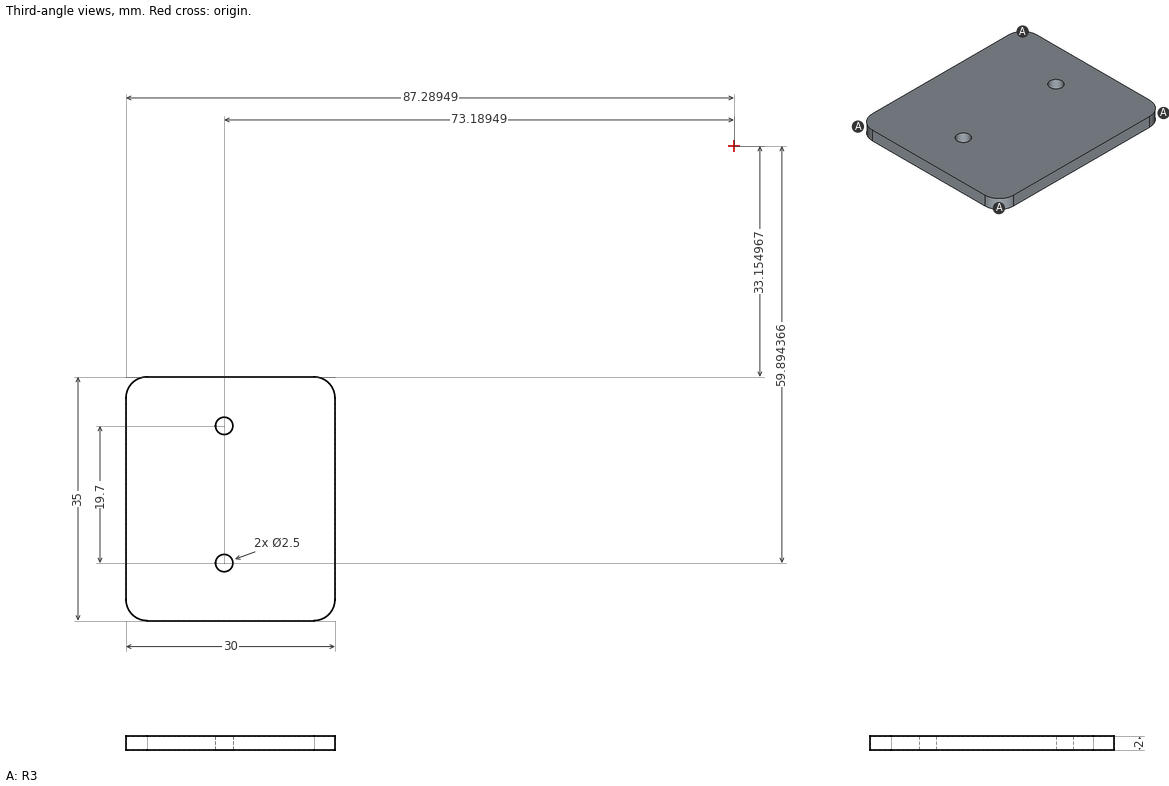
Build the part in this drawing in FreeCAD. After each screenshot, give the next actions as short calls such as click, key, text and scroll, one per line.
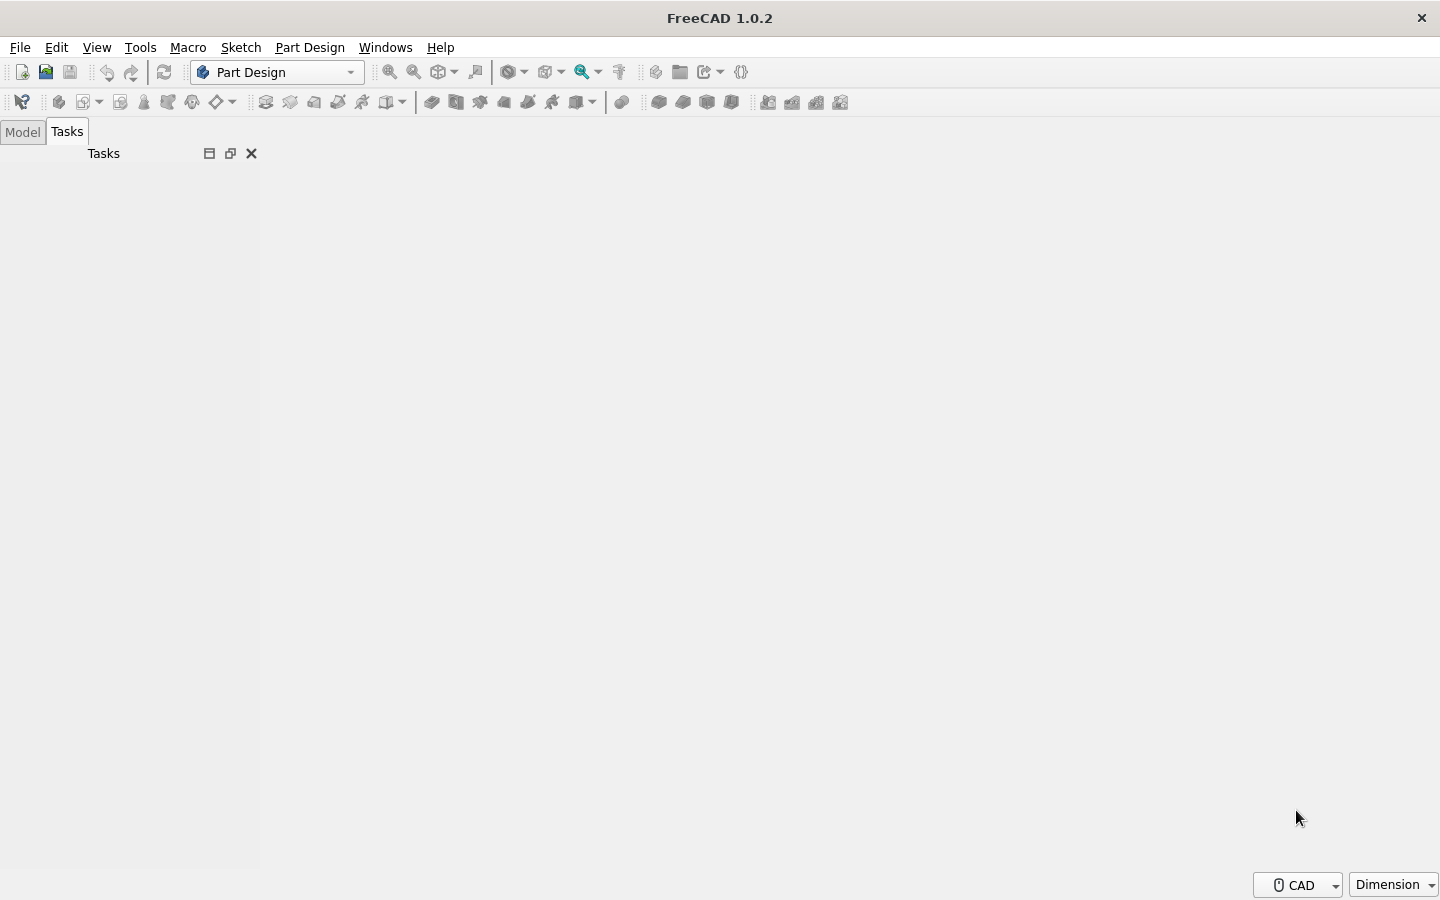
click(22, 72)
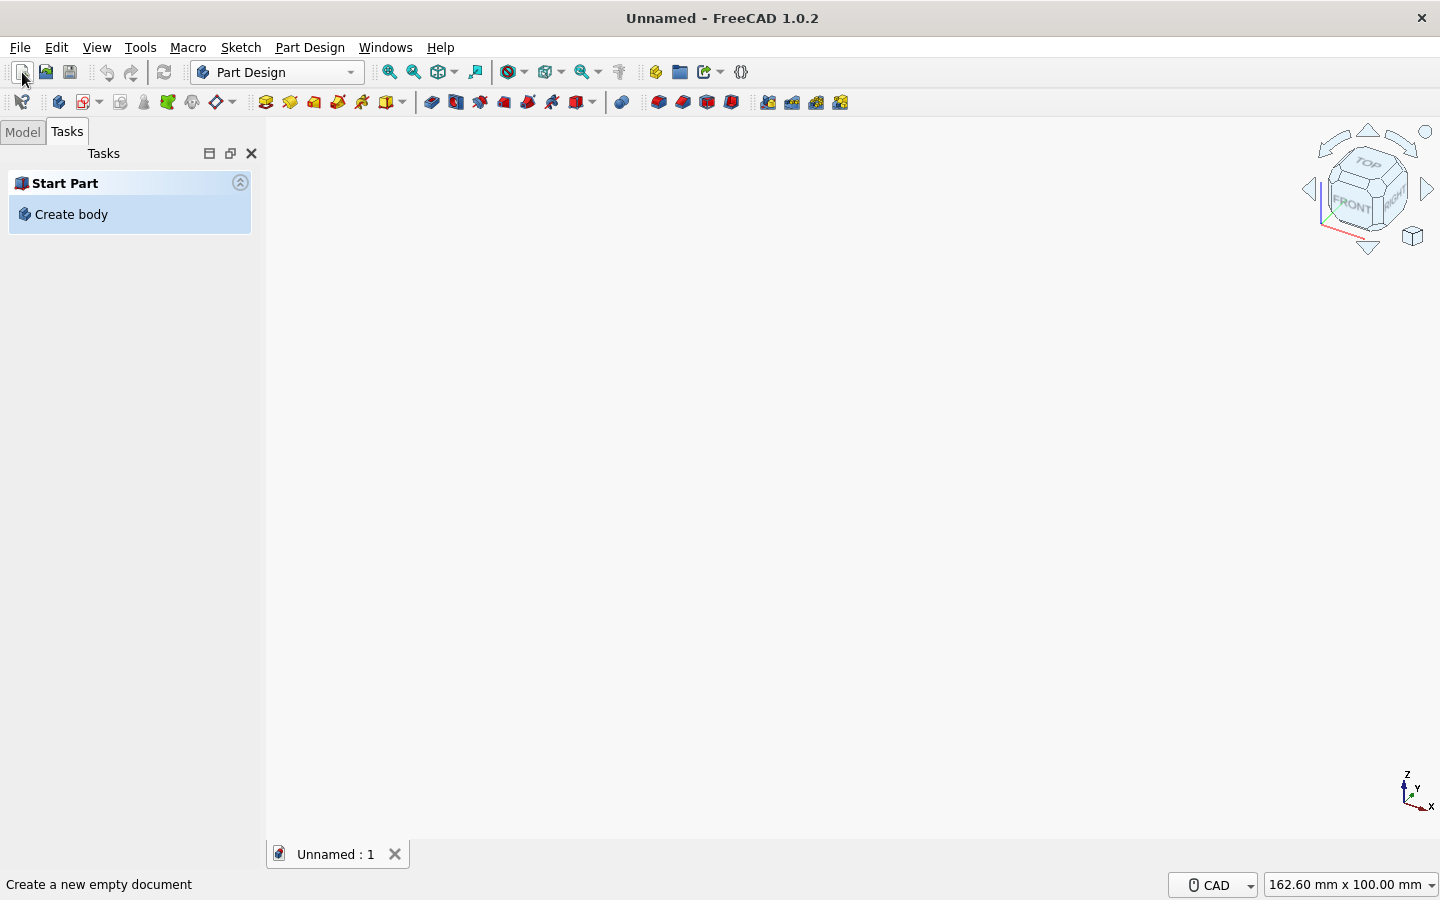
click(84, 102)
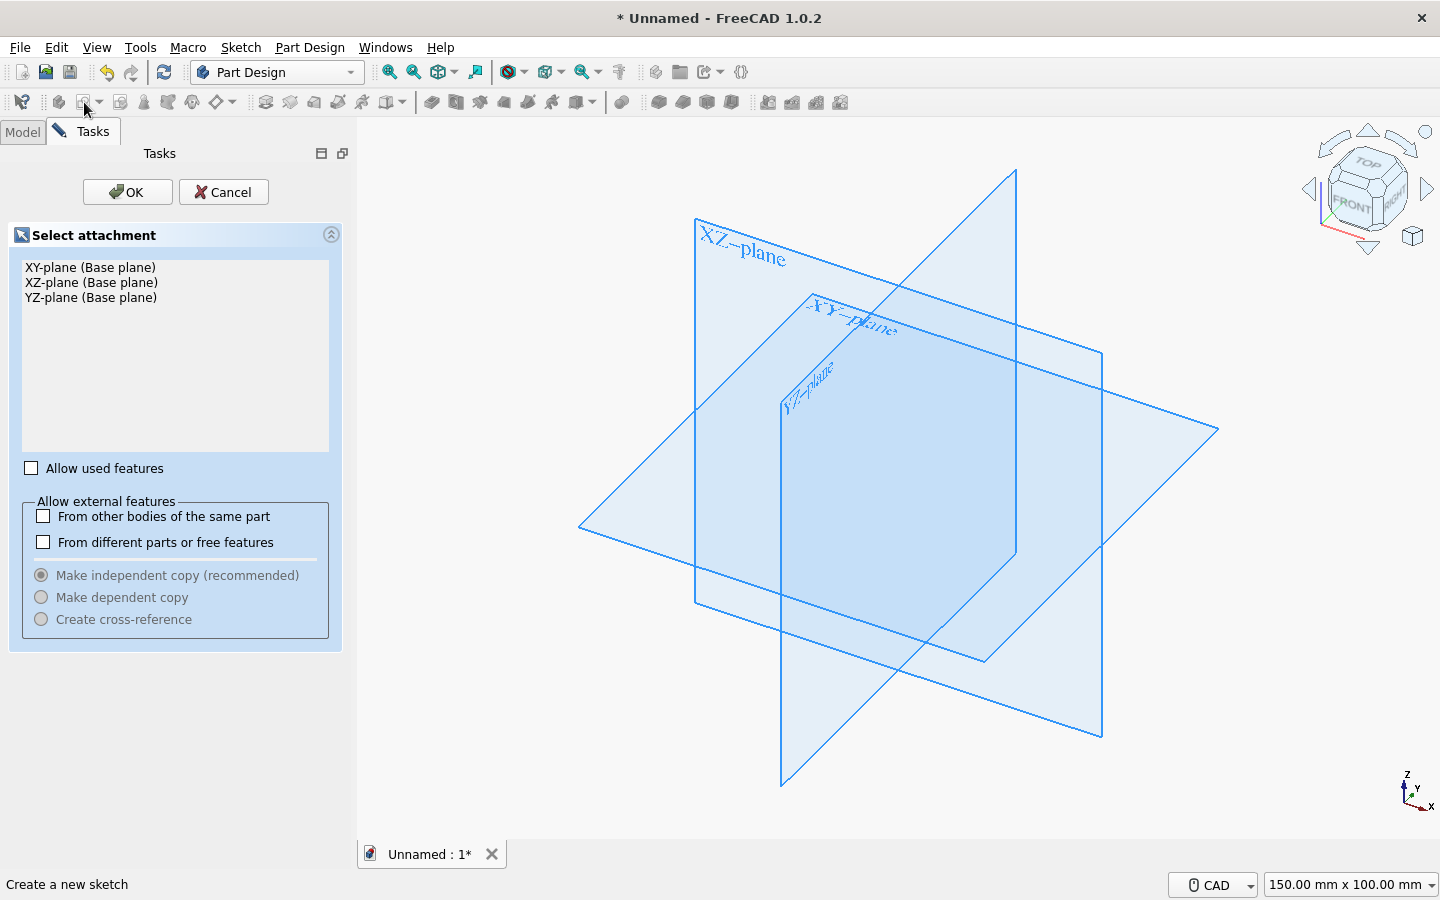
click(82, 268)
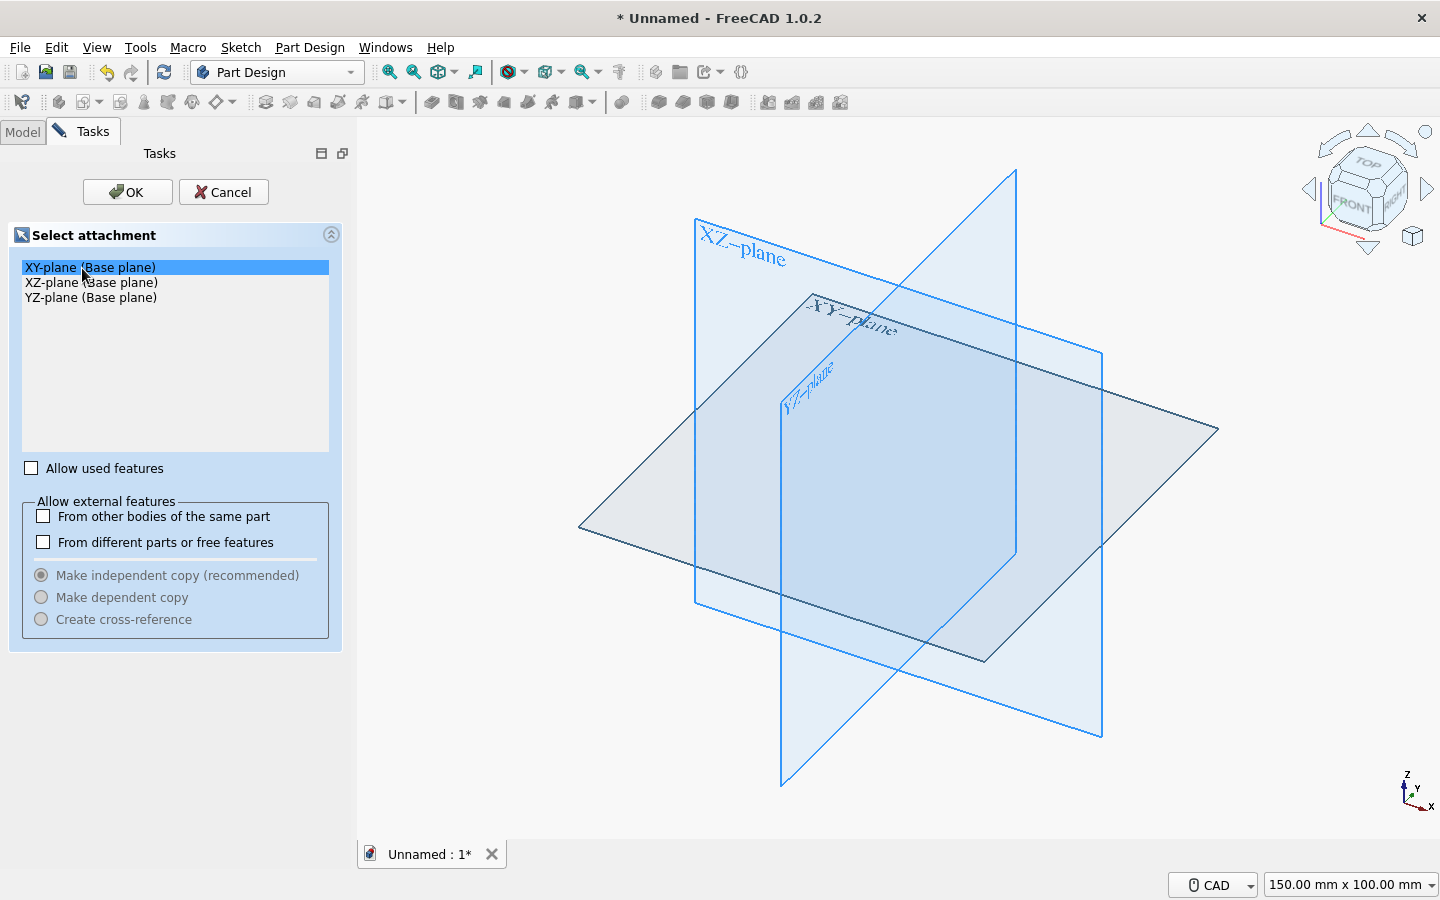
click(128, 192)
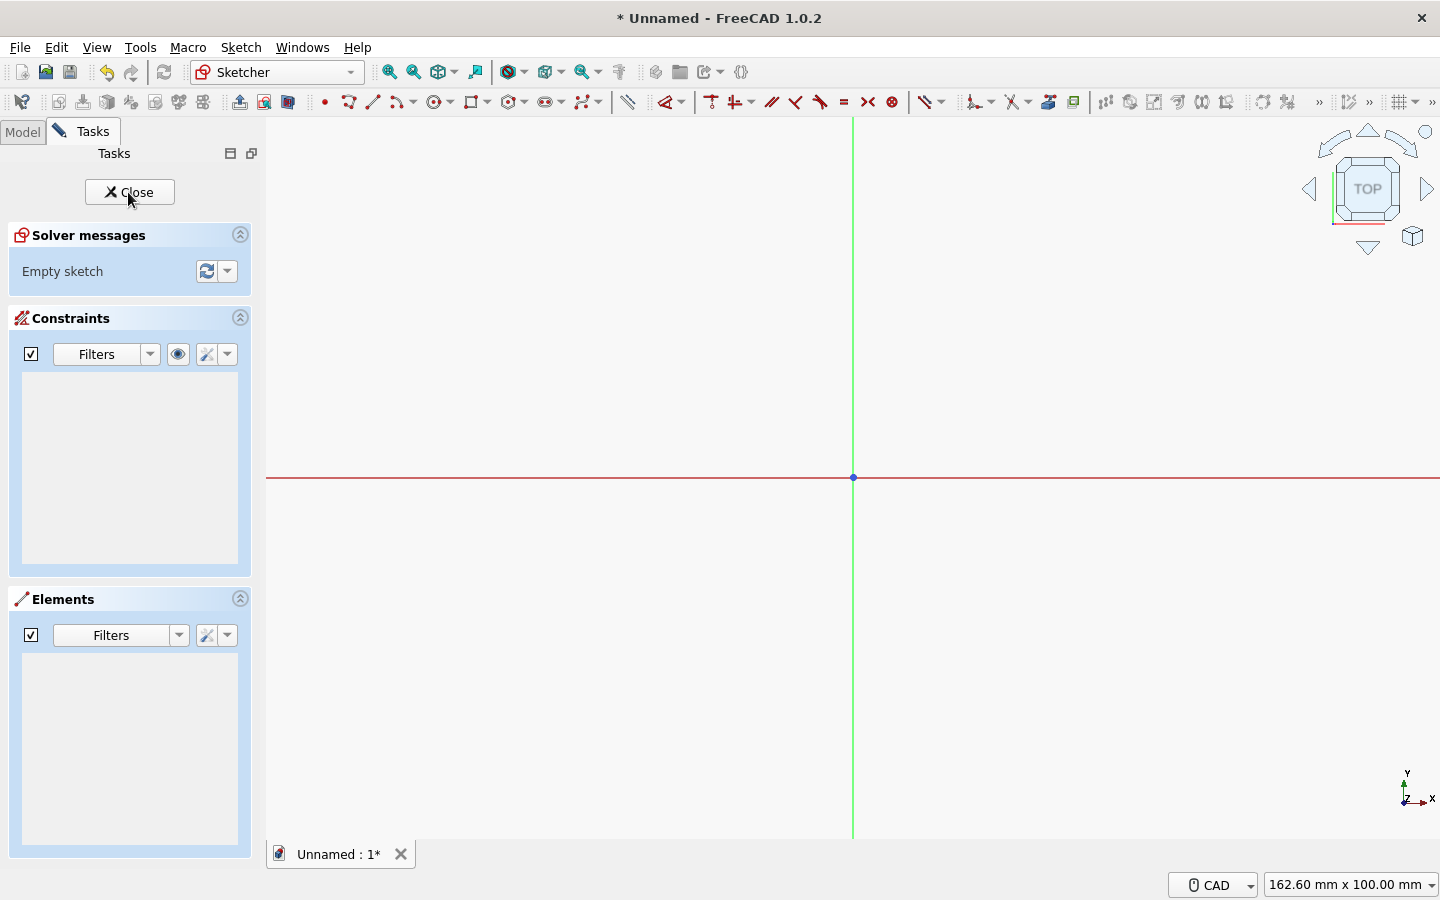
scroll(1275, 145, down, 2)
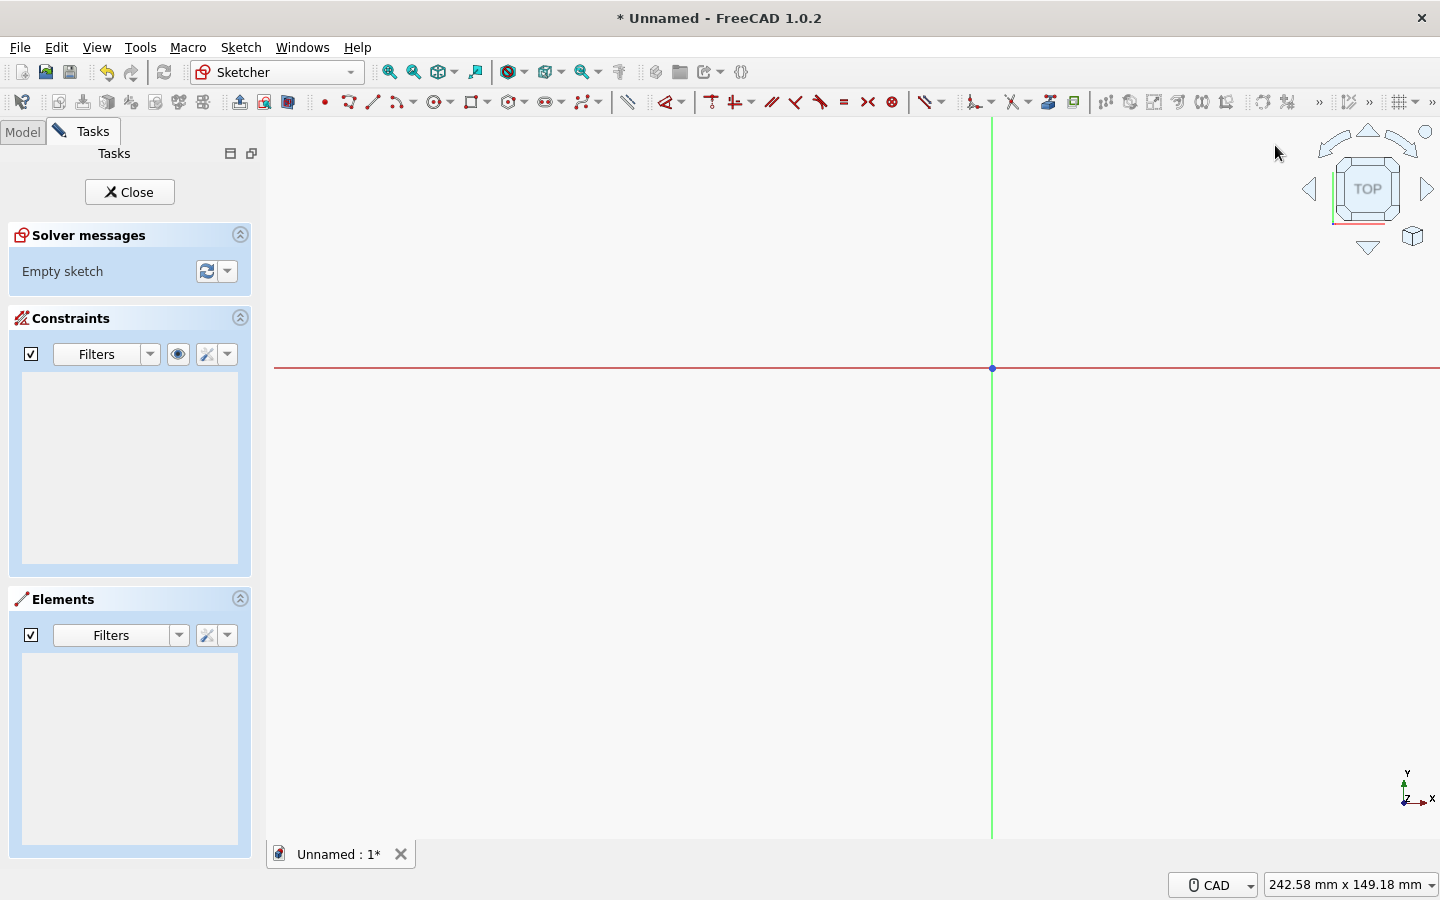
scroll(774, 645, up, 2)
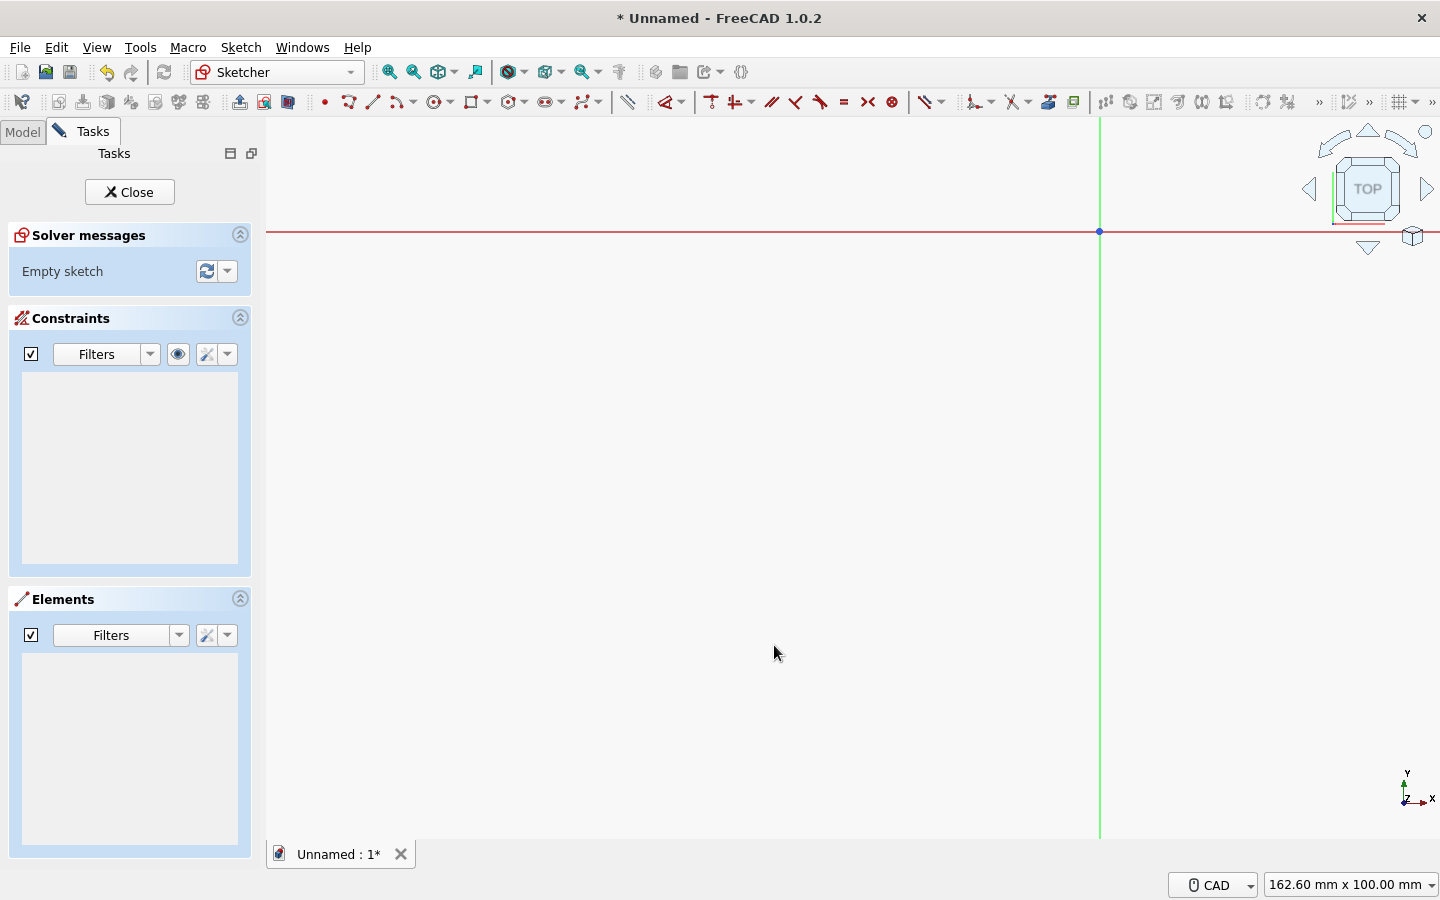
click(472, 102)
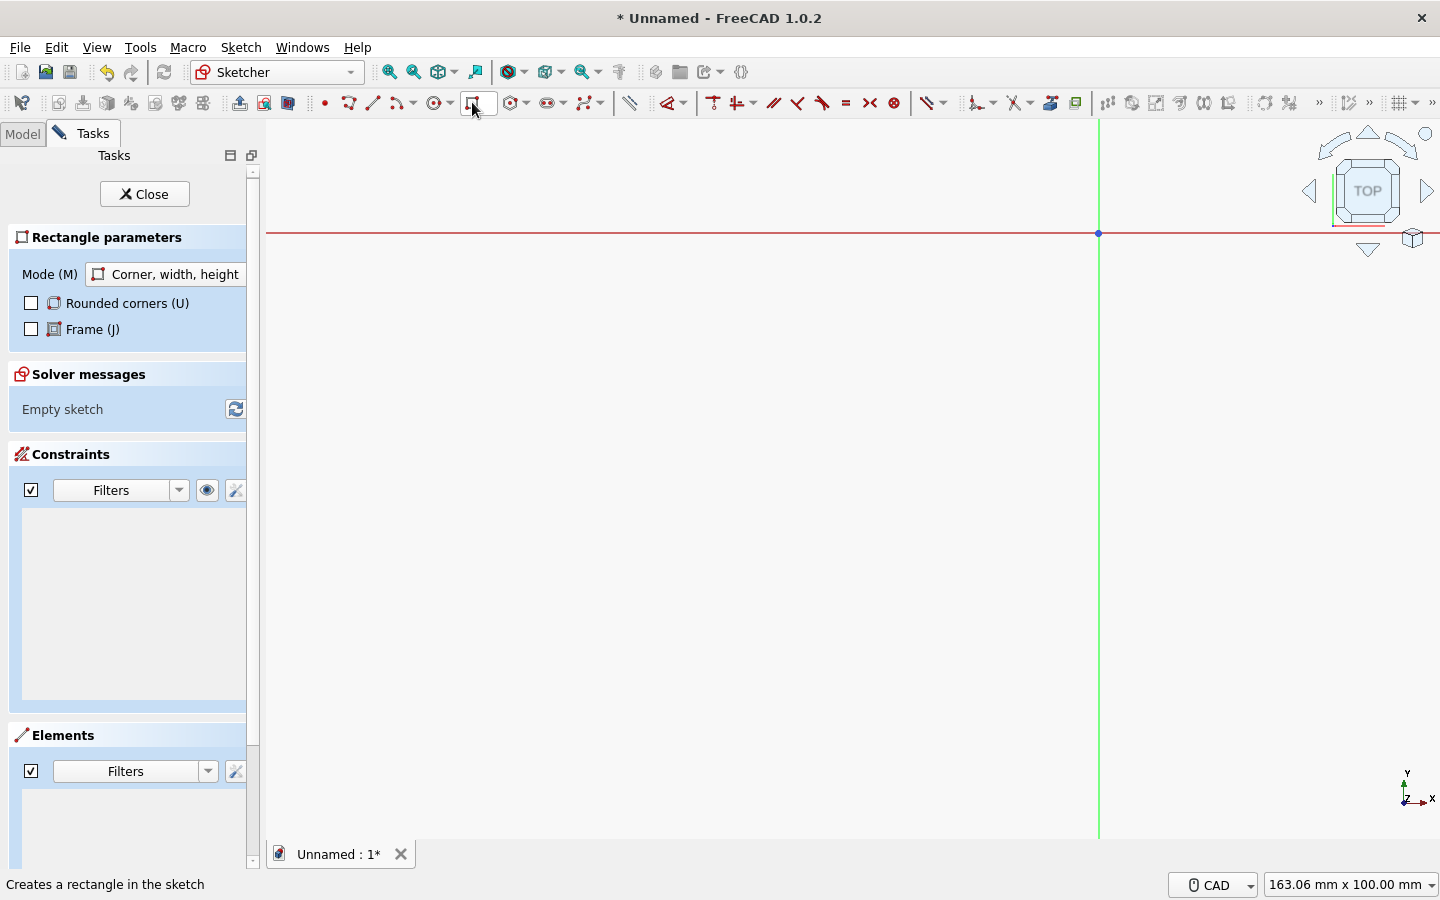
click(470, 472)
move(686, 724)